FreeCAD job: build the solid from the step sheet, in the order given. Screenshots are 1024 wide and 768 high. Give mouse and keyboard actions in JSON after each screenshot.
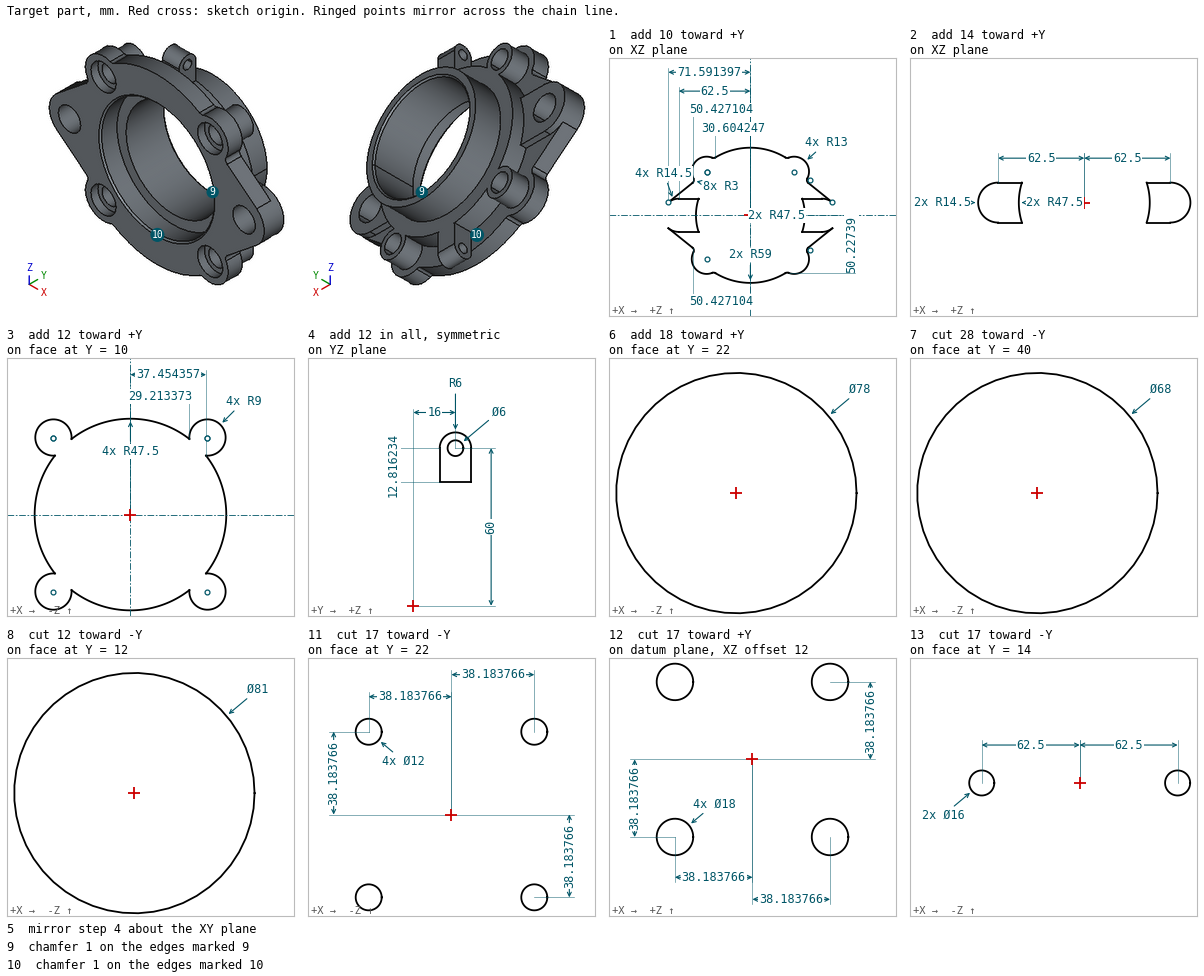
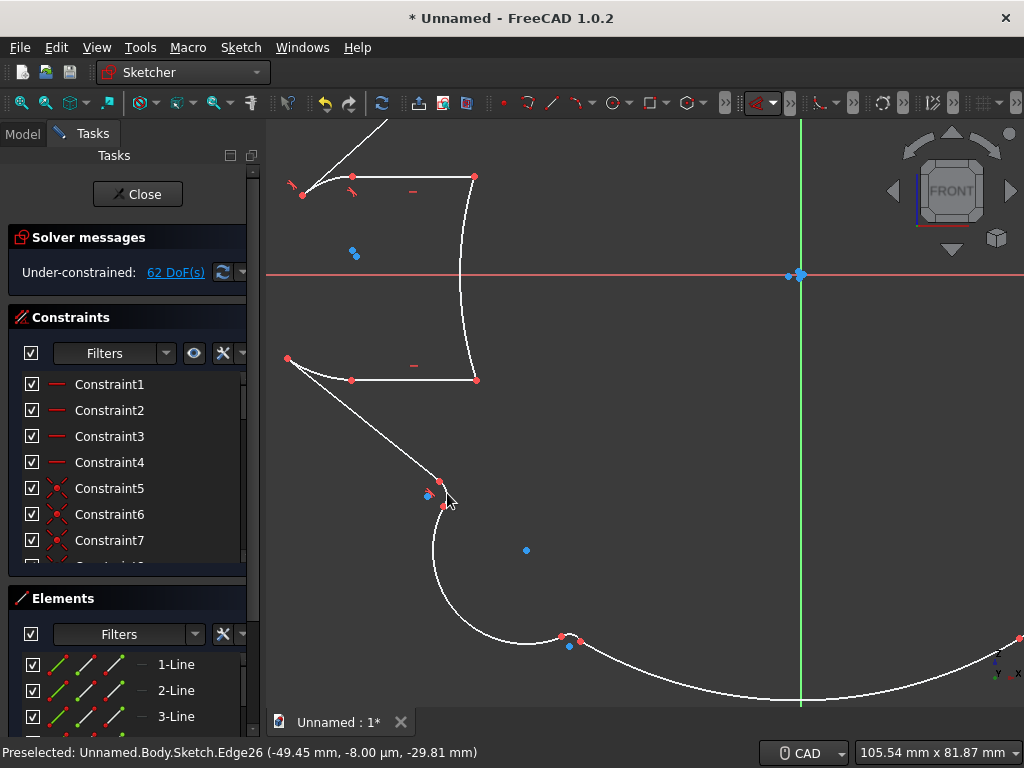
{"action": "left_click", "coordinate": [394, 444]}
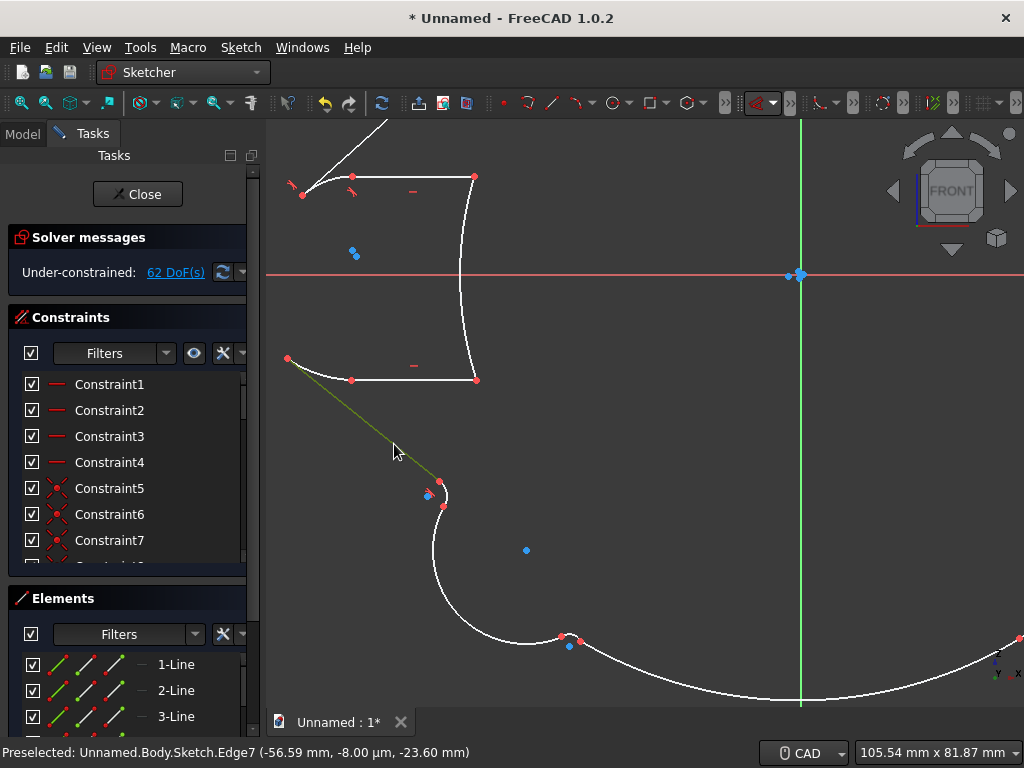
{"action": "left_click", "coordinate": [331, 377]}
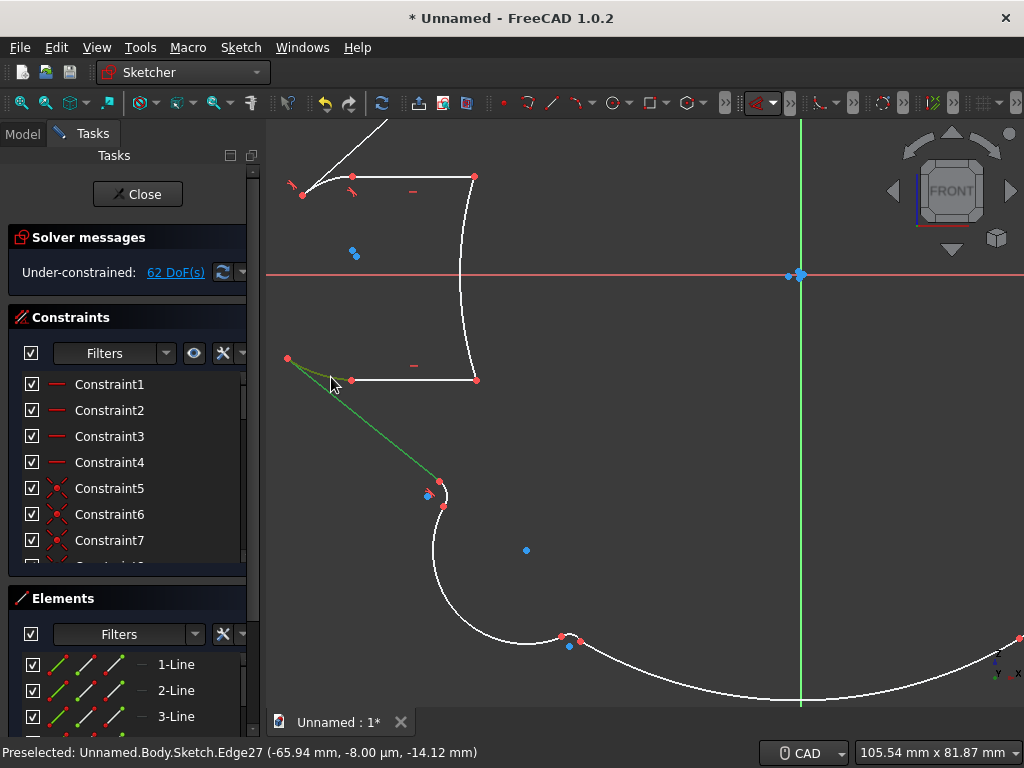
{"action": "key", "text": "t"}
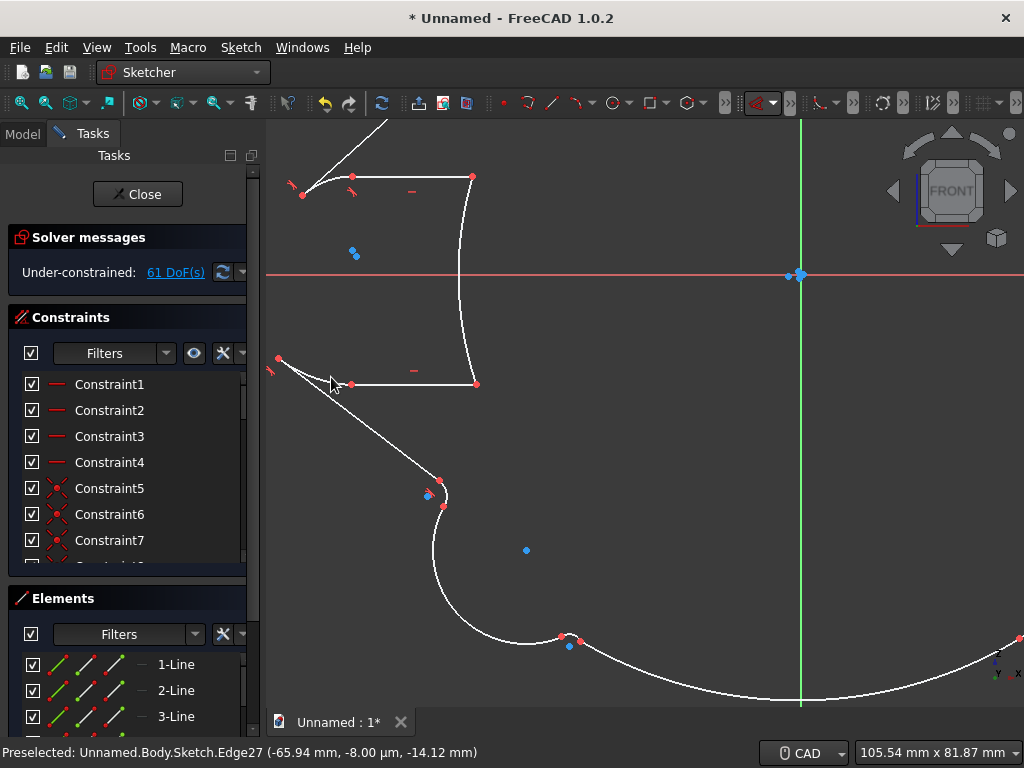
{"action": "left_click", "coordinate": [389, 385]}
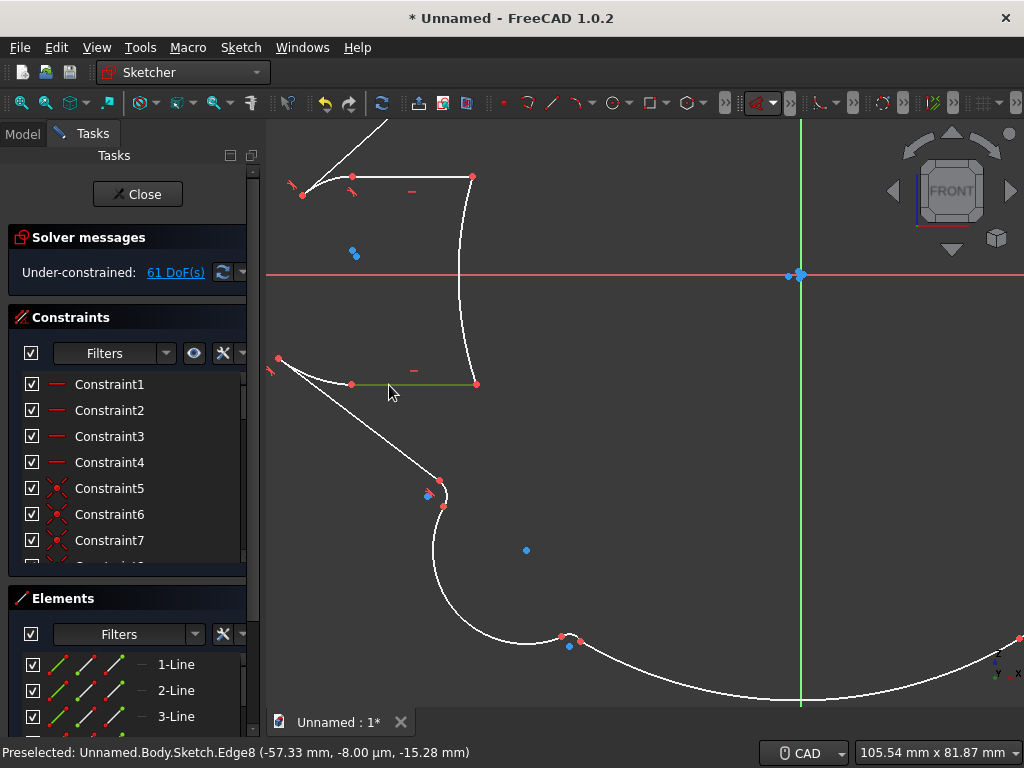
{"action": "left_click", "coordinate": [328, 382]}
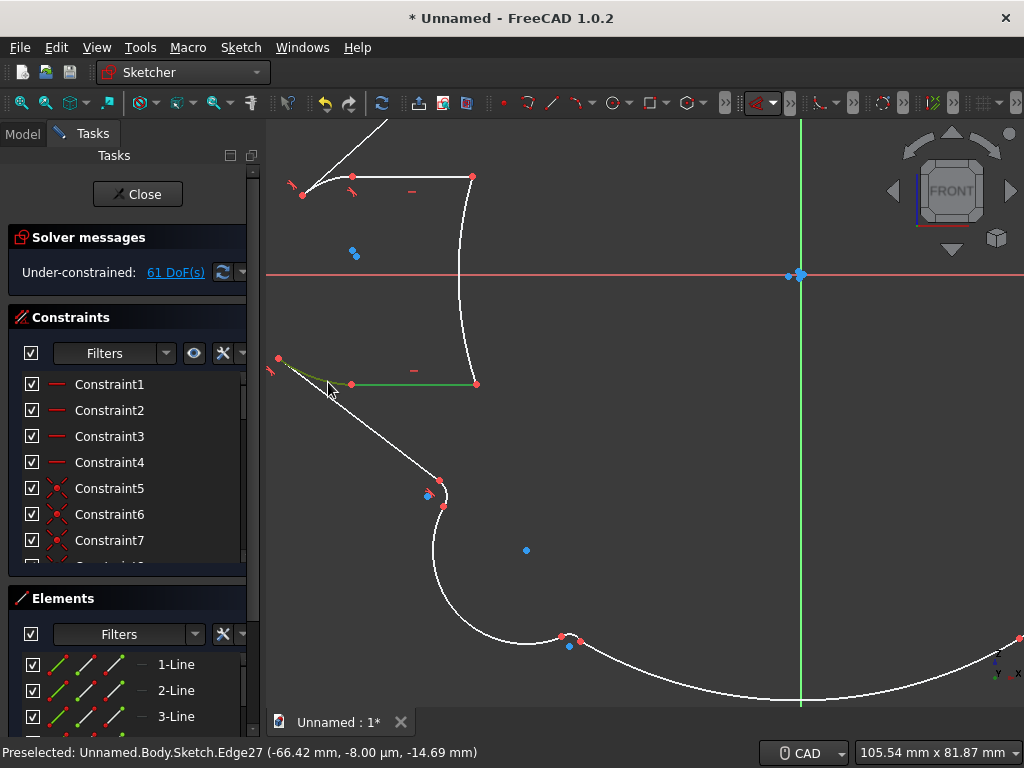
{"action": "key", "text": "t"}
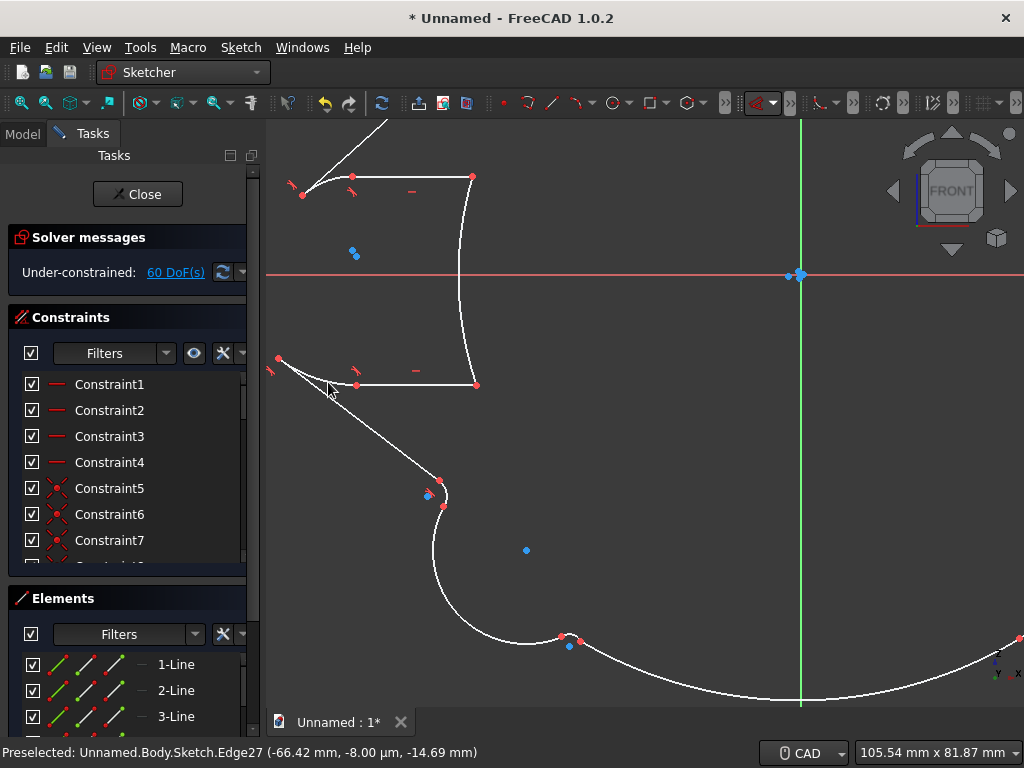
{"action": "scroll", "coordinate": [446, 493], "scroll_direction": "down", "scroll_amount": 5}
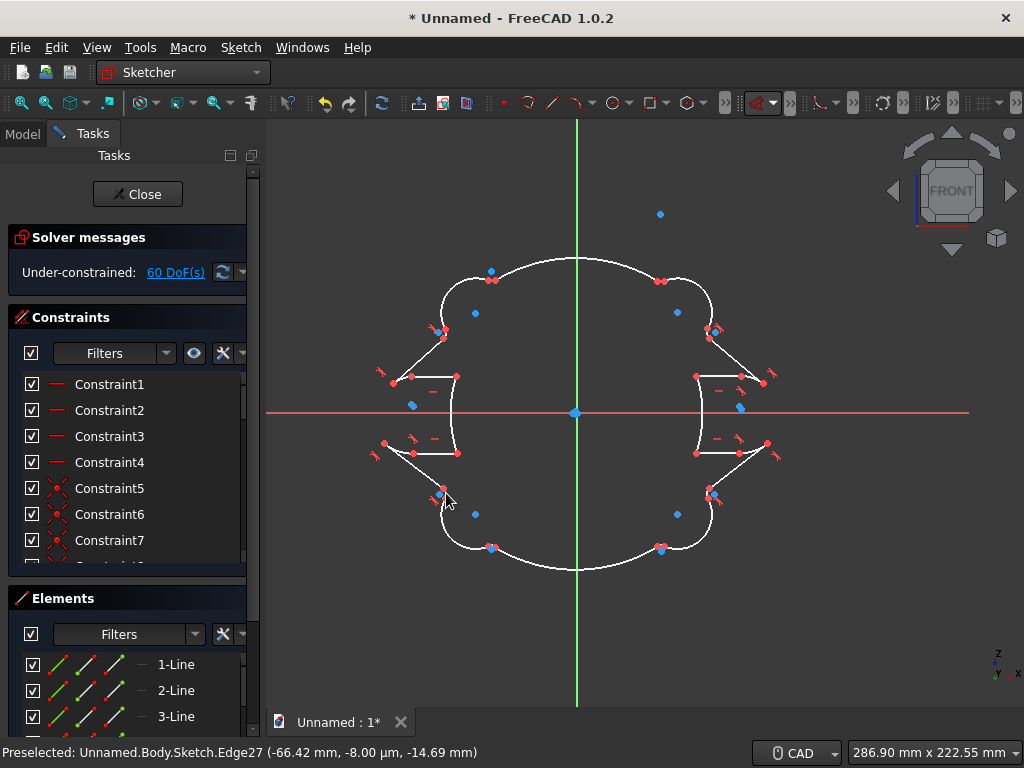
{"action": "scroll", "coordinate": [446, 334], "scroll_direction": "up", "scroll_amount": 5}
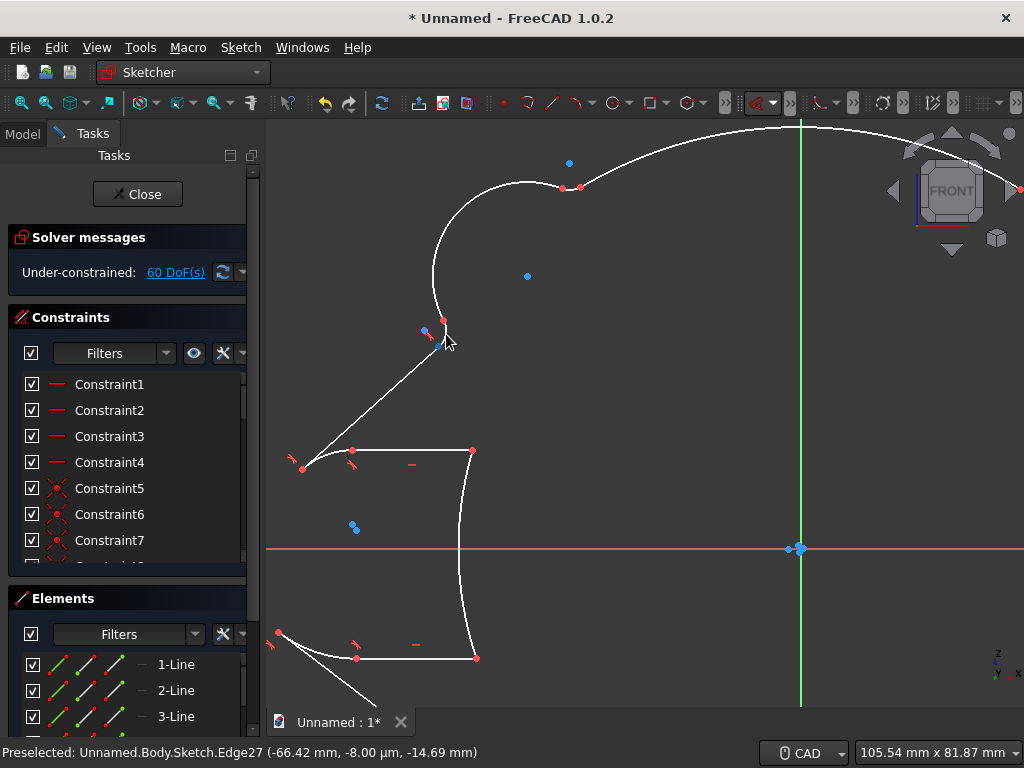
{"action": "left_click", "coordinate": [446, 334]}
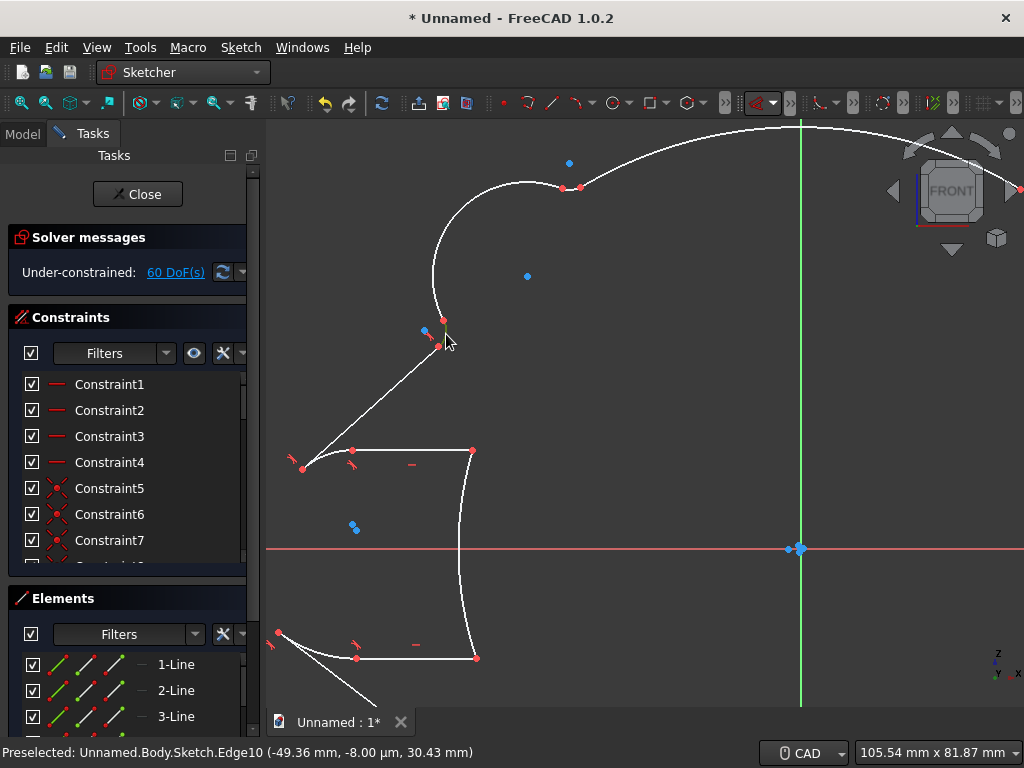
{"action": "left_click", "coordinate": [495, 188]}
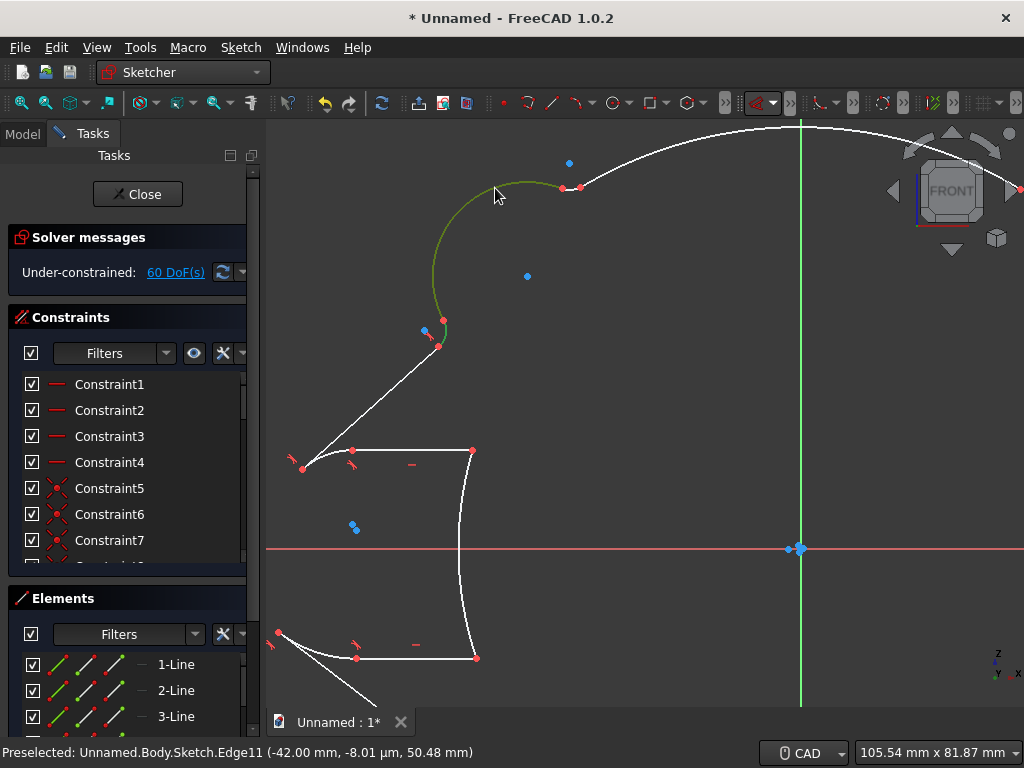
{"action": "key", "text": "t"}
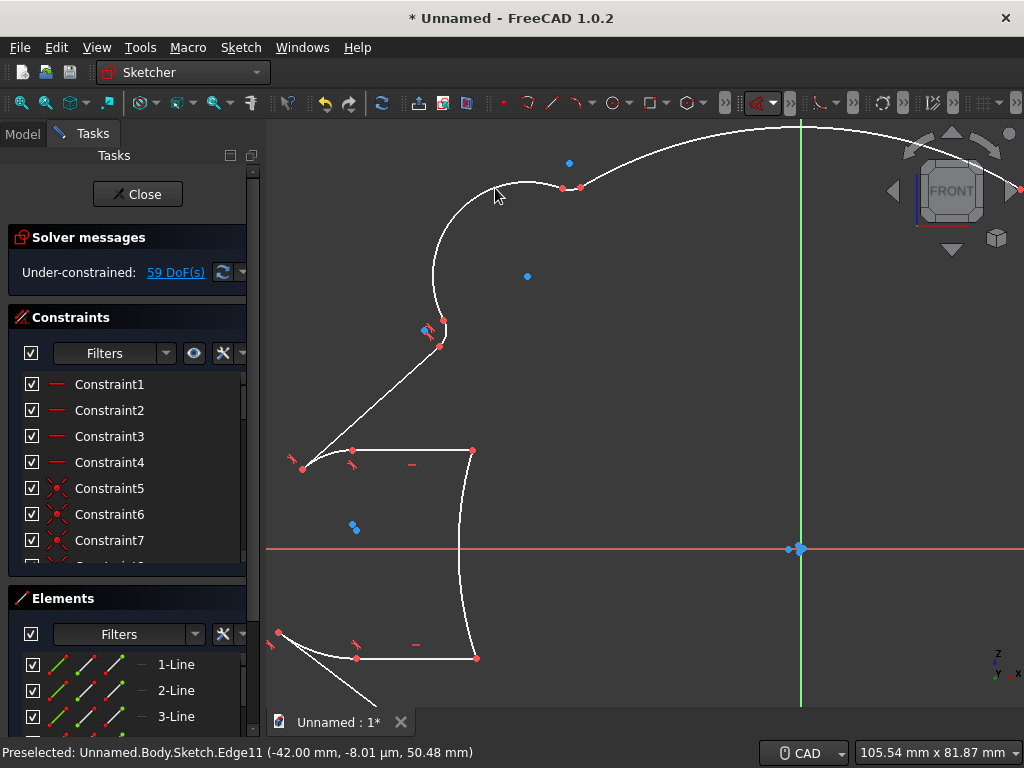
{"action": "left_click", "coordinate": [495, 188]}